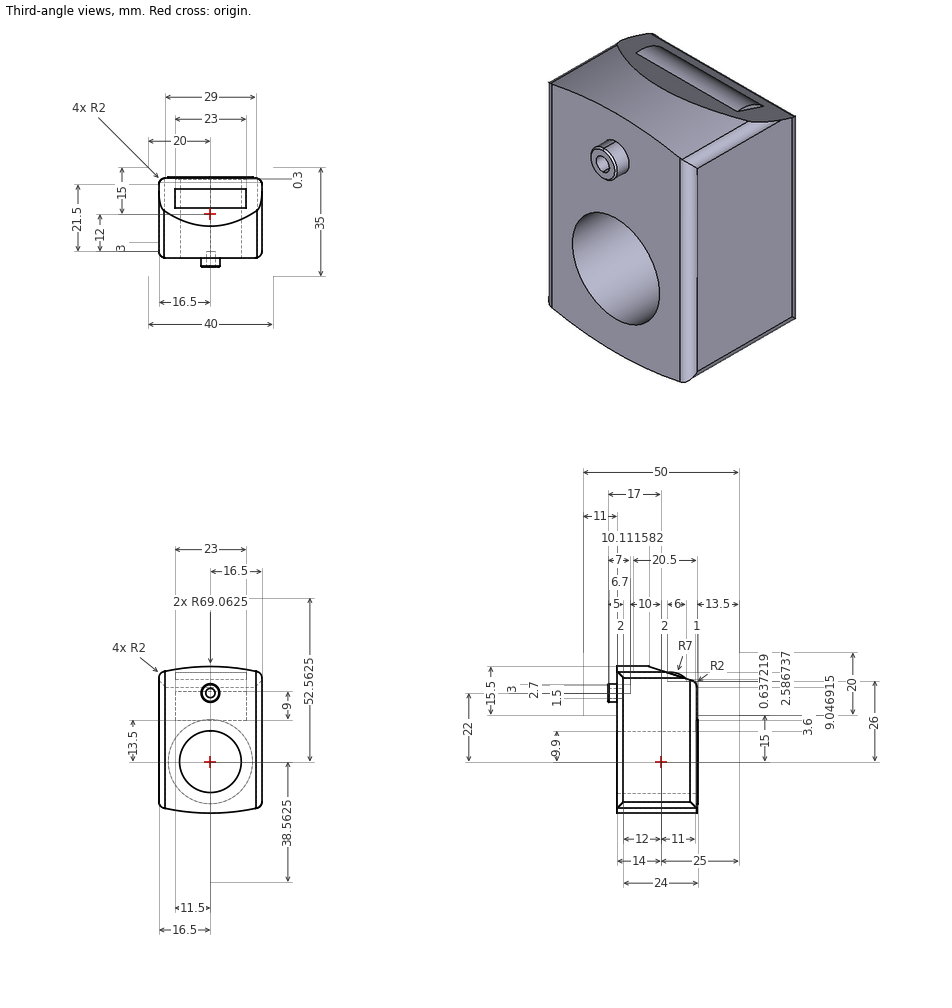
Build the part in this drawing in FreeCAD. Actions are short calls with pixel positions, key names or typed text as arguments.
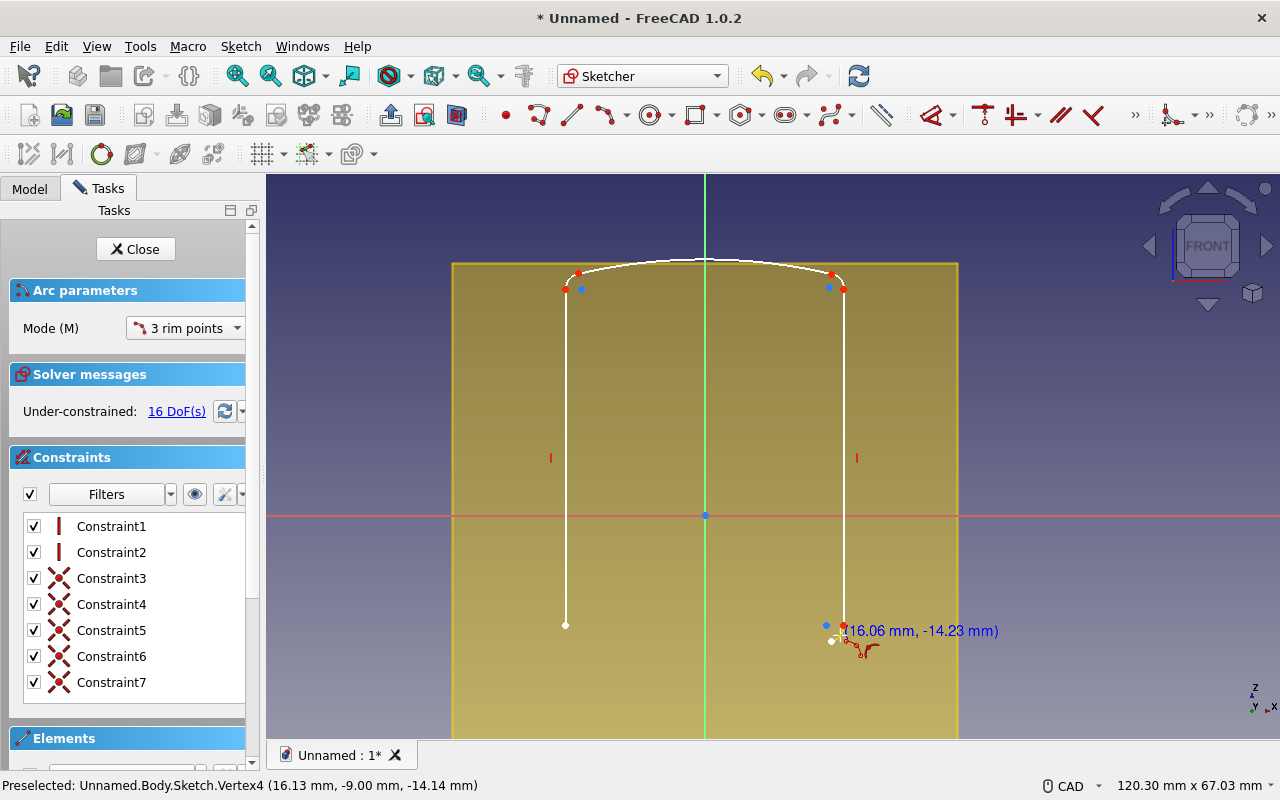
click(831, 642)
click(579, 641)
click(680, 654)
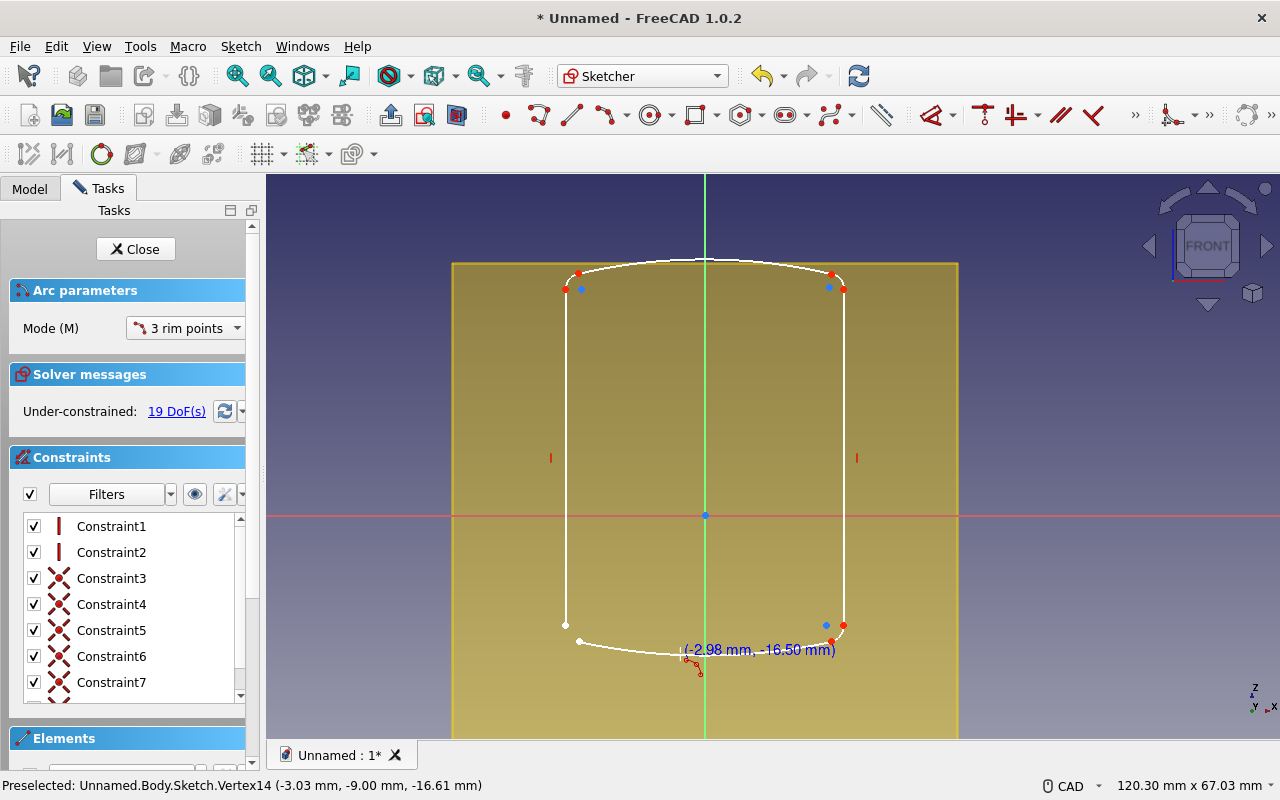
click(579, 642)
click(566, 626)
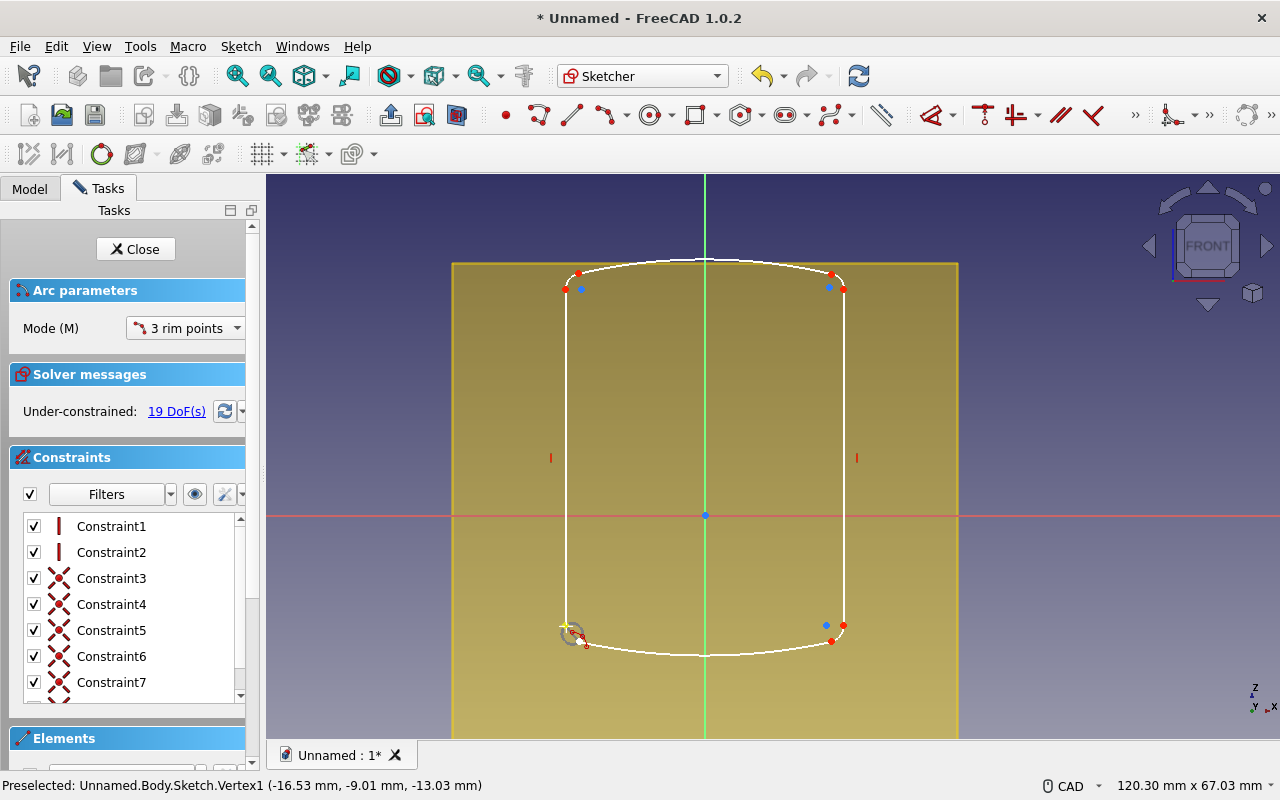
scroll(570, 635, up, 8)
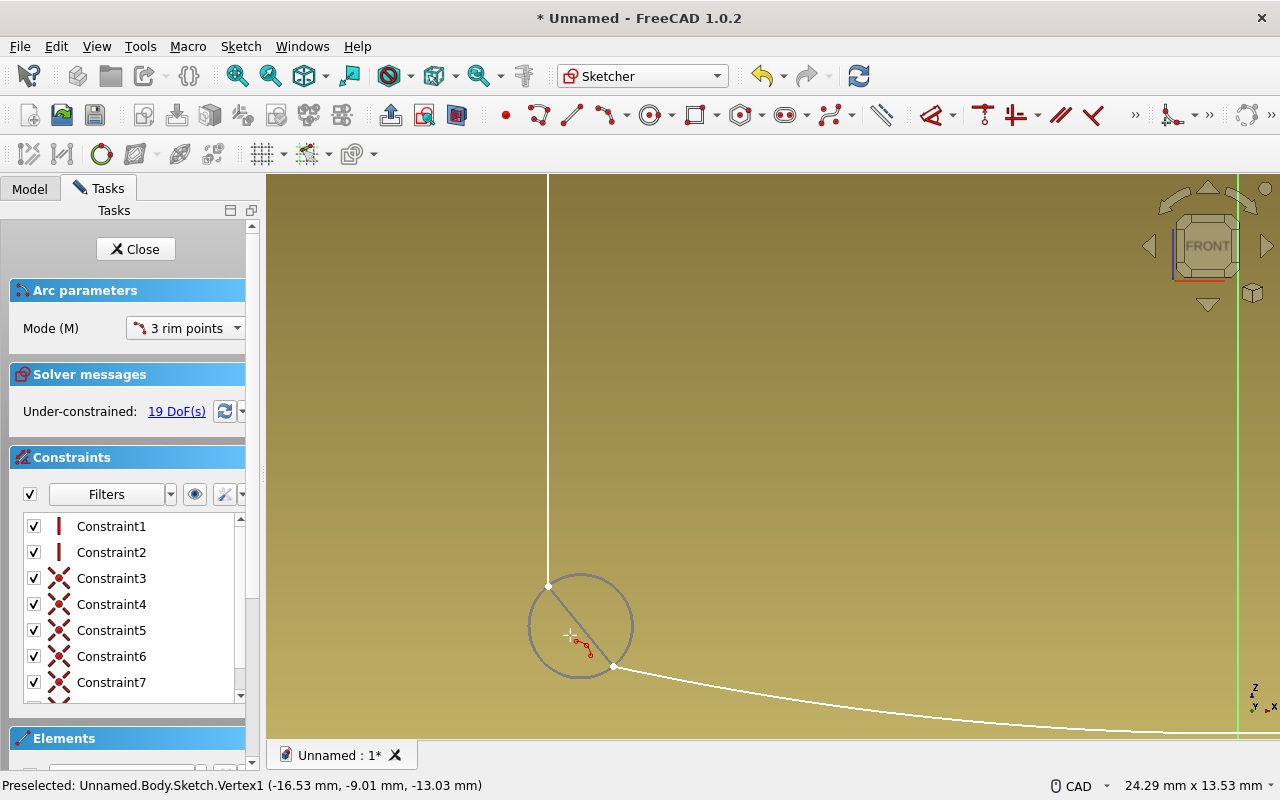
click(568, 633)
key(Escape)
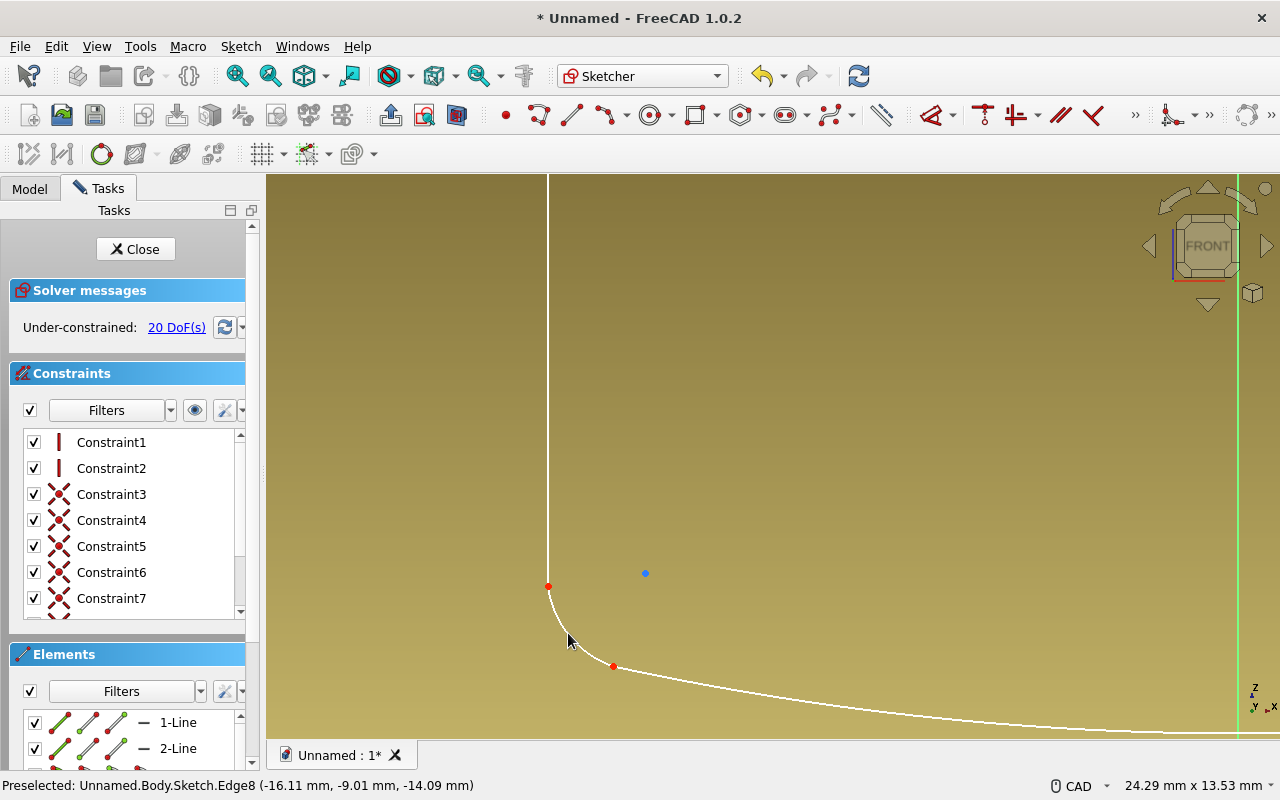
scroll(570, 635, down, 8)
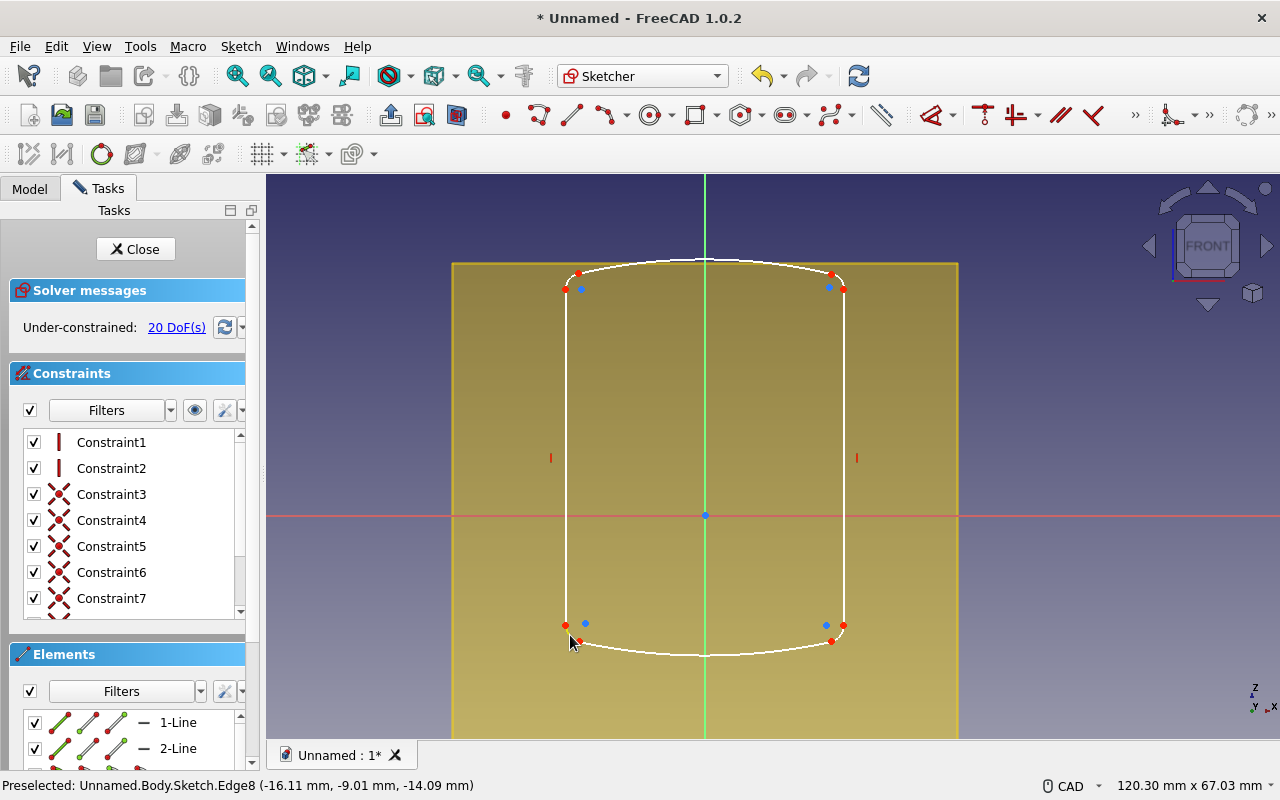
click(566, 559)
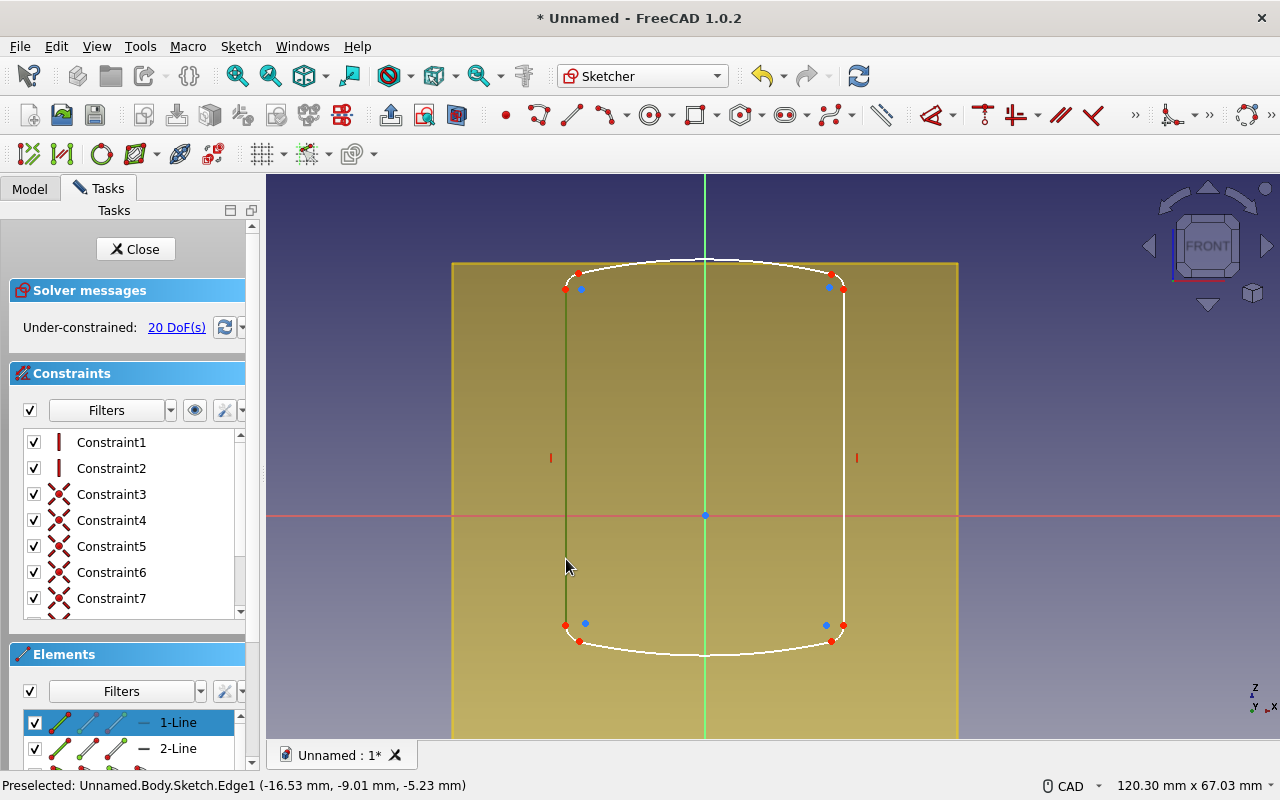
scroll(569, 279, up, 2)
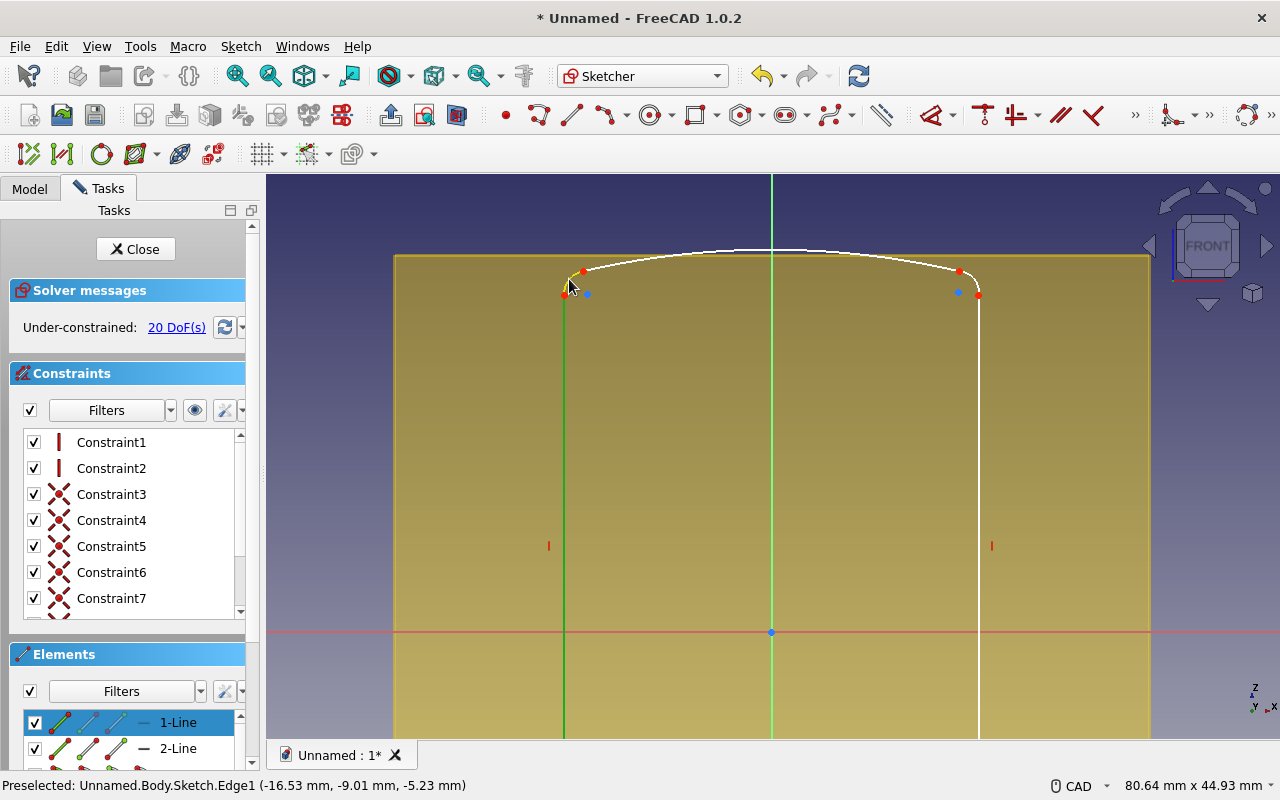
click(569, 279)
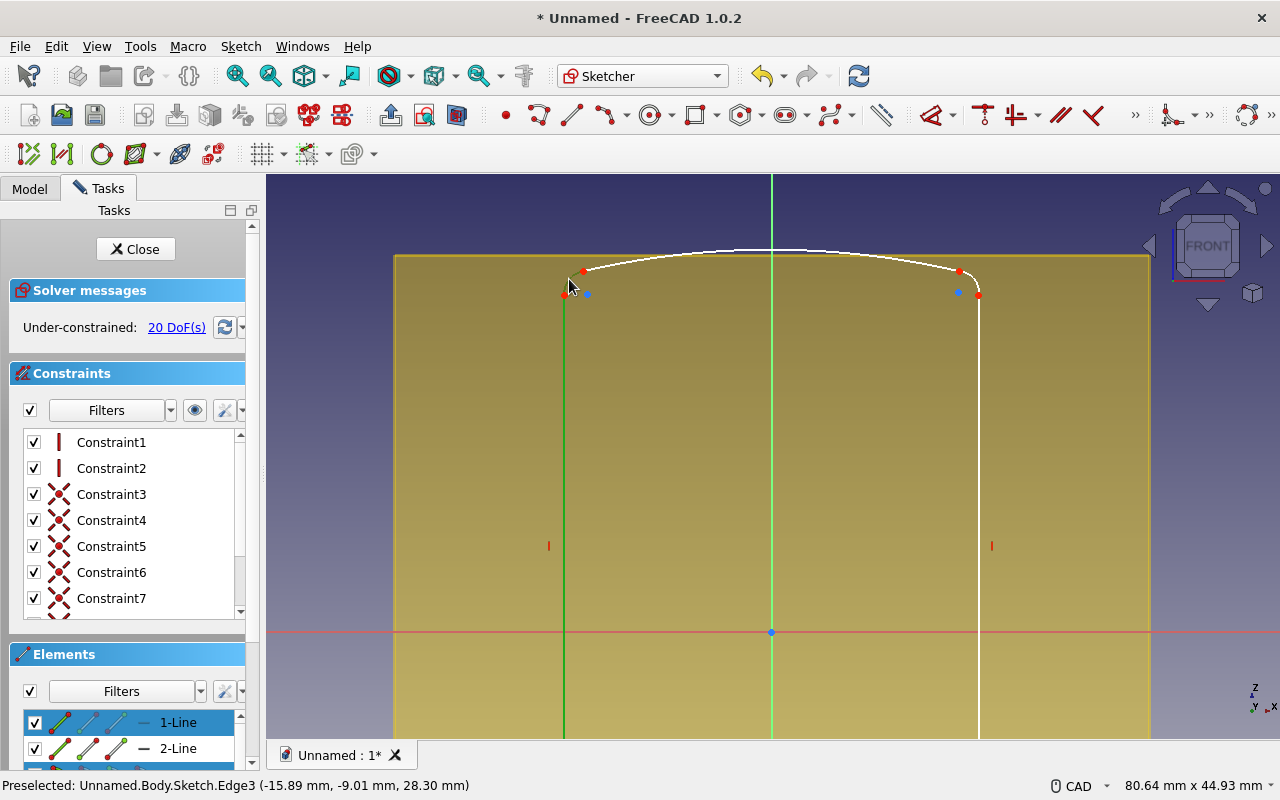
key(t)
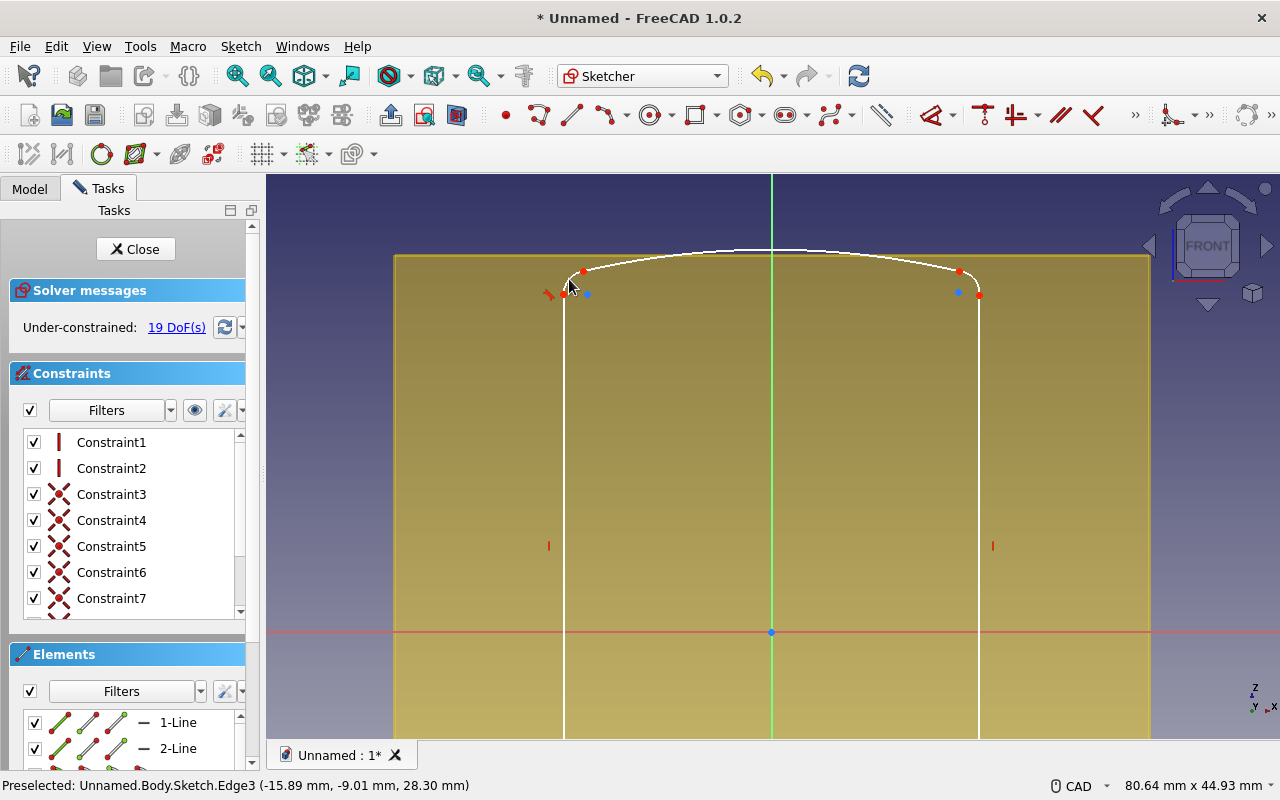
click(564, 646)